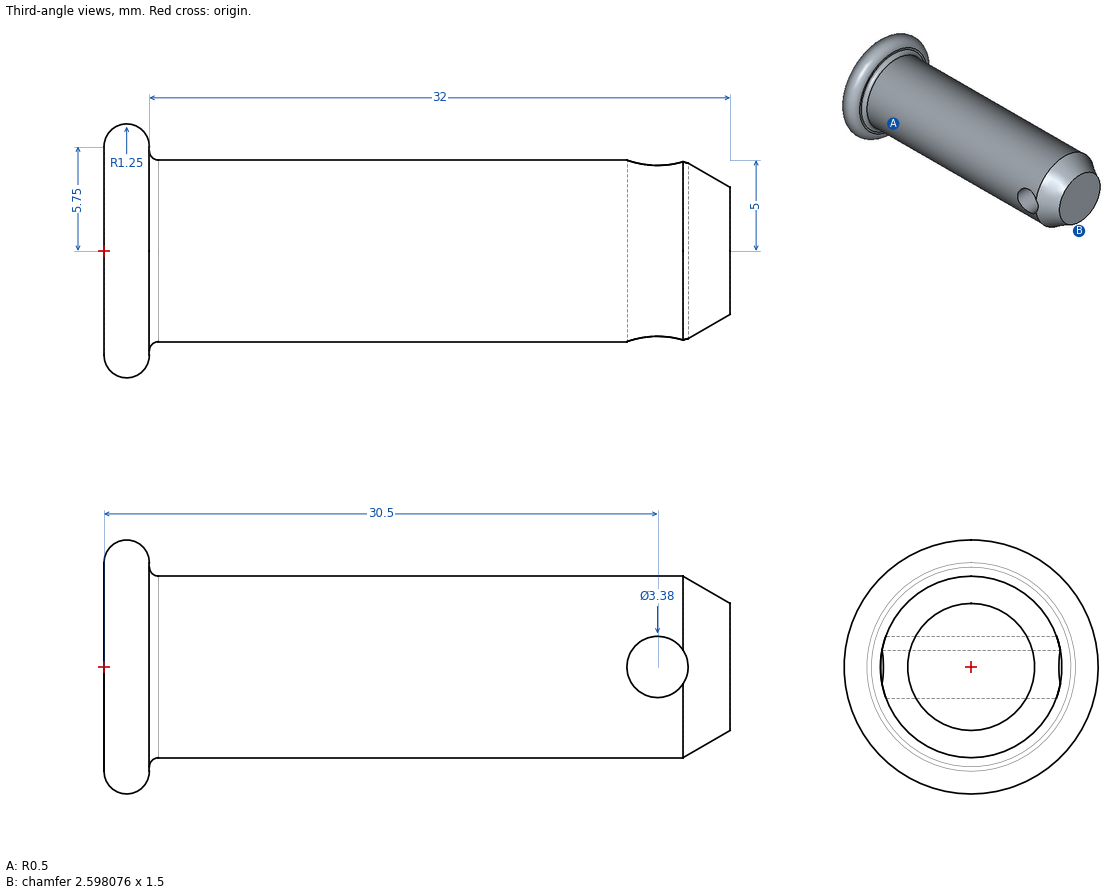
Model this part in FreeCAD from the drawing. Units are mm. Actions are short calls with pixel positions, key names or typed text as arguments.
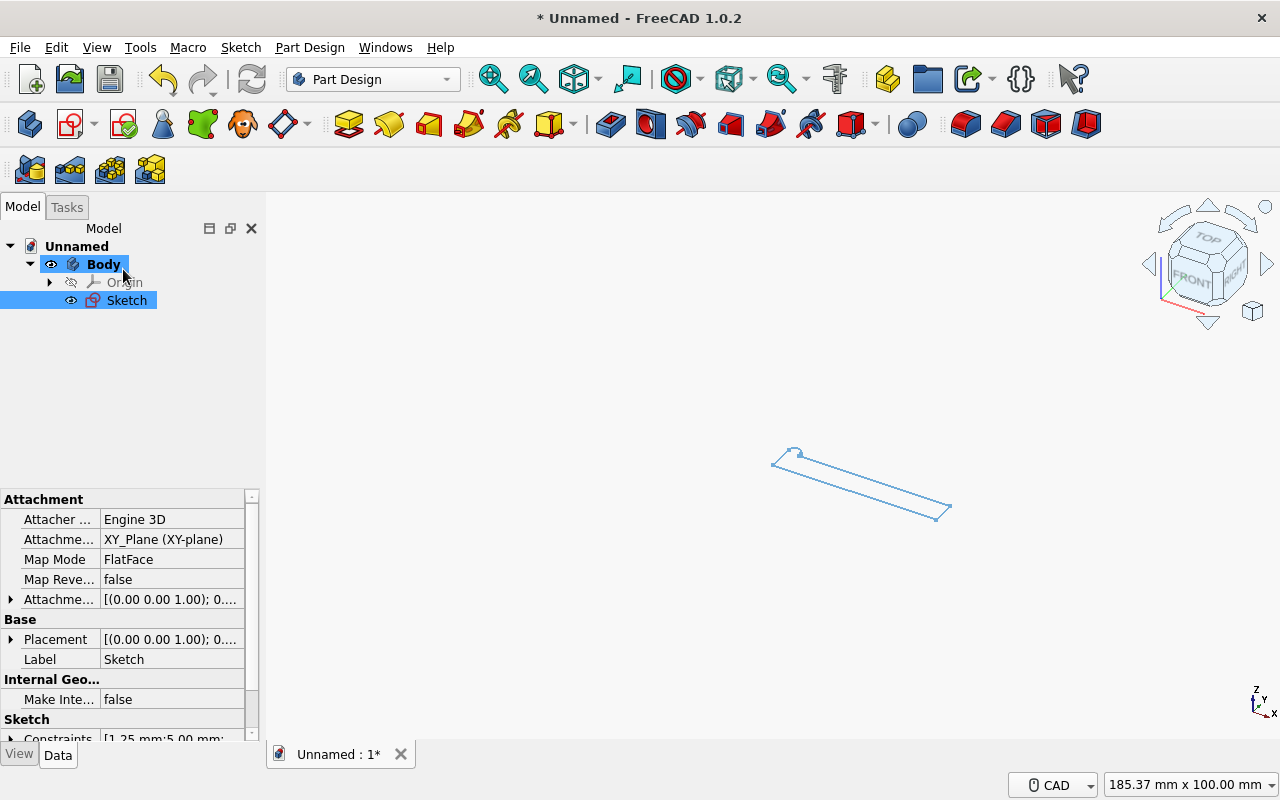
click(390, 124)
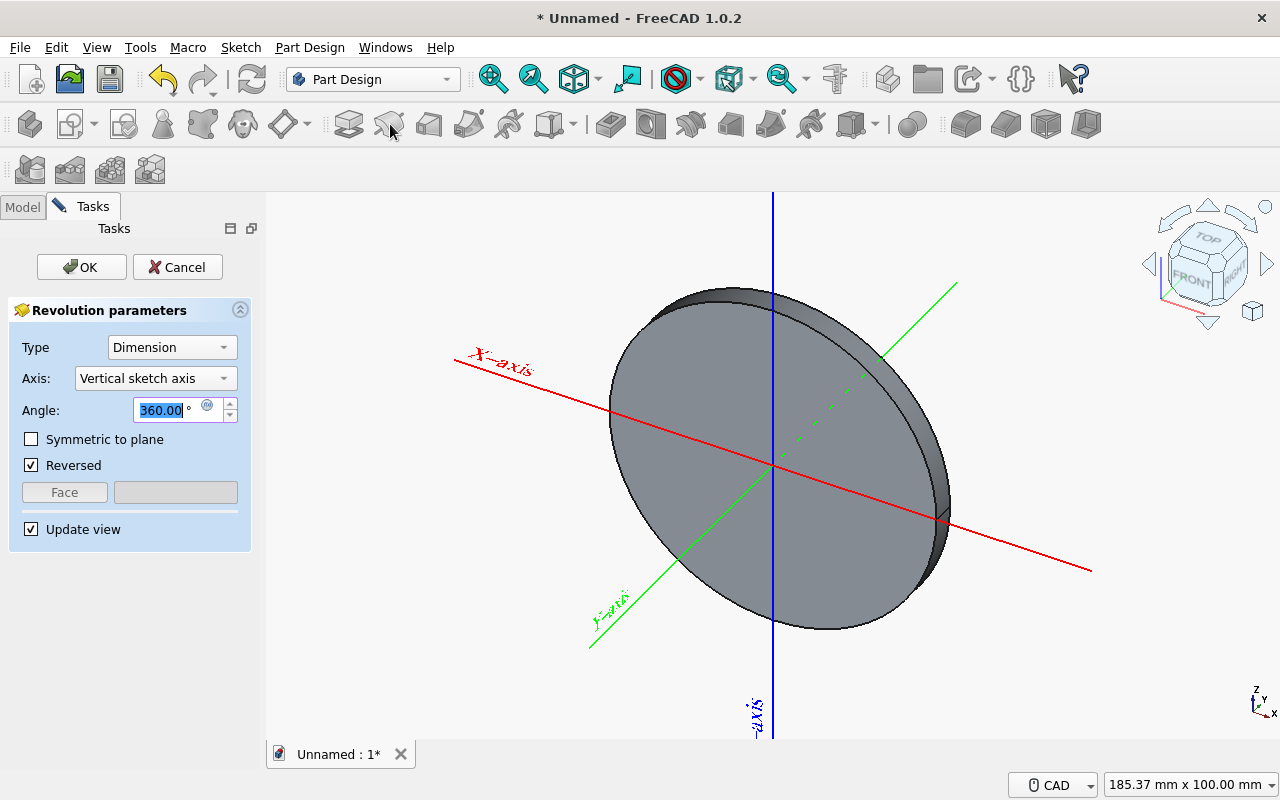
click(156, 378)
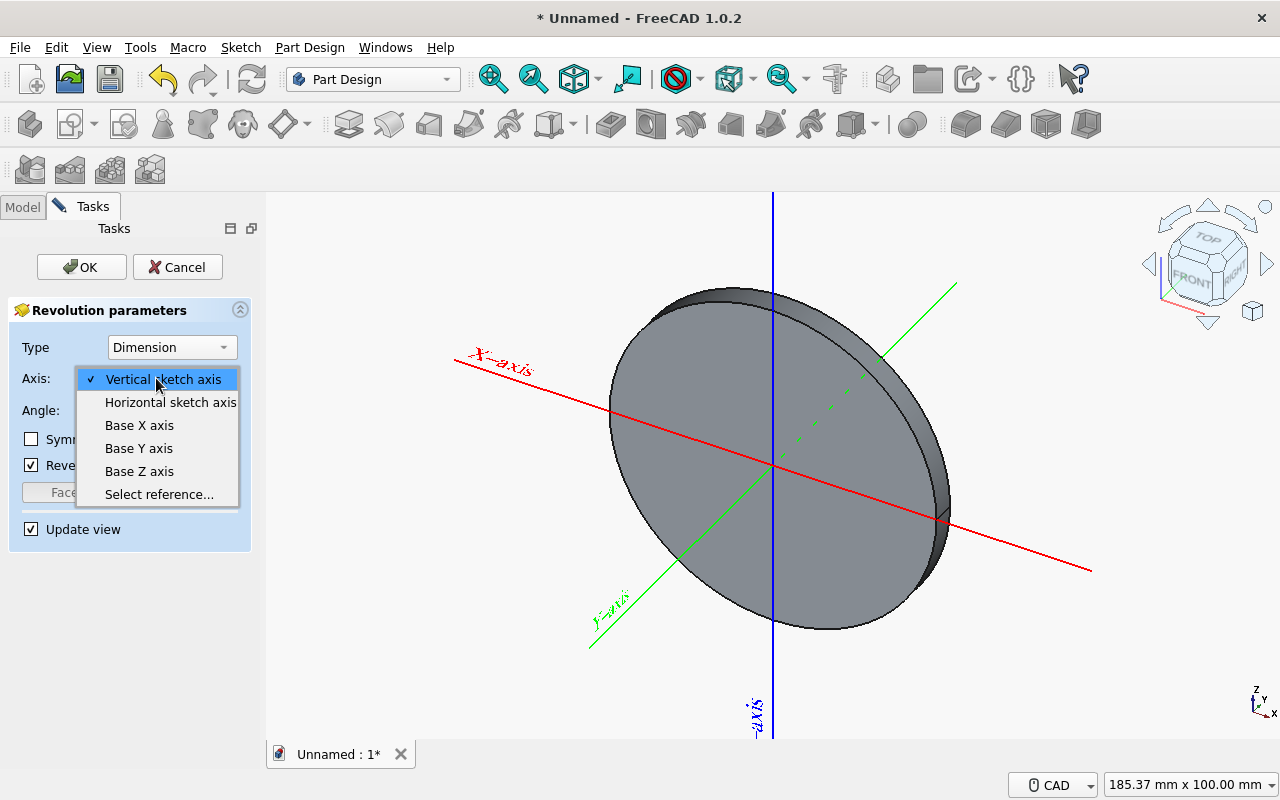
click(156, 402)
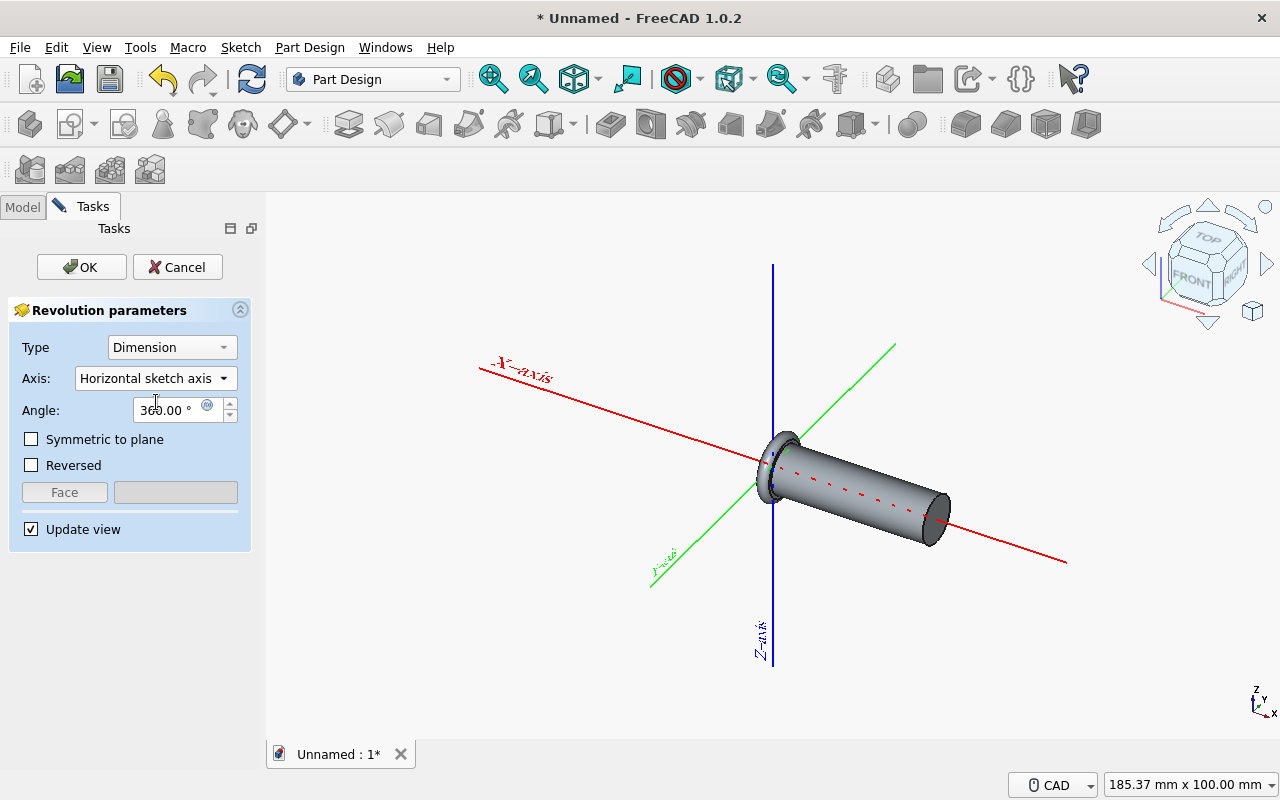
click(82, 267)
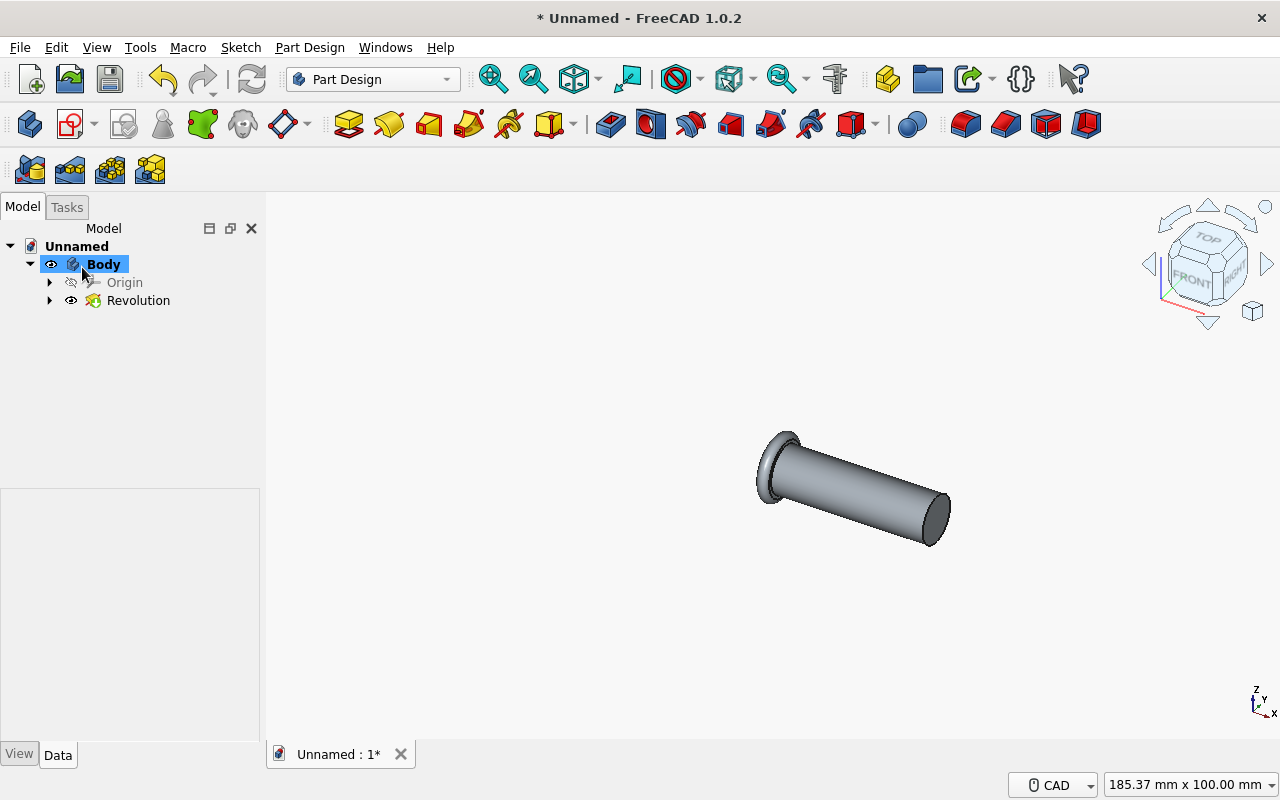
click(494, 80)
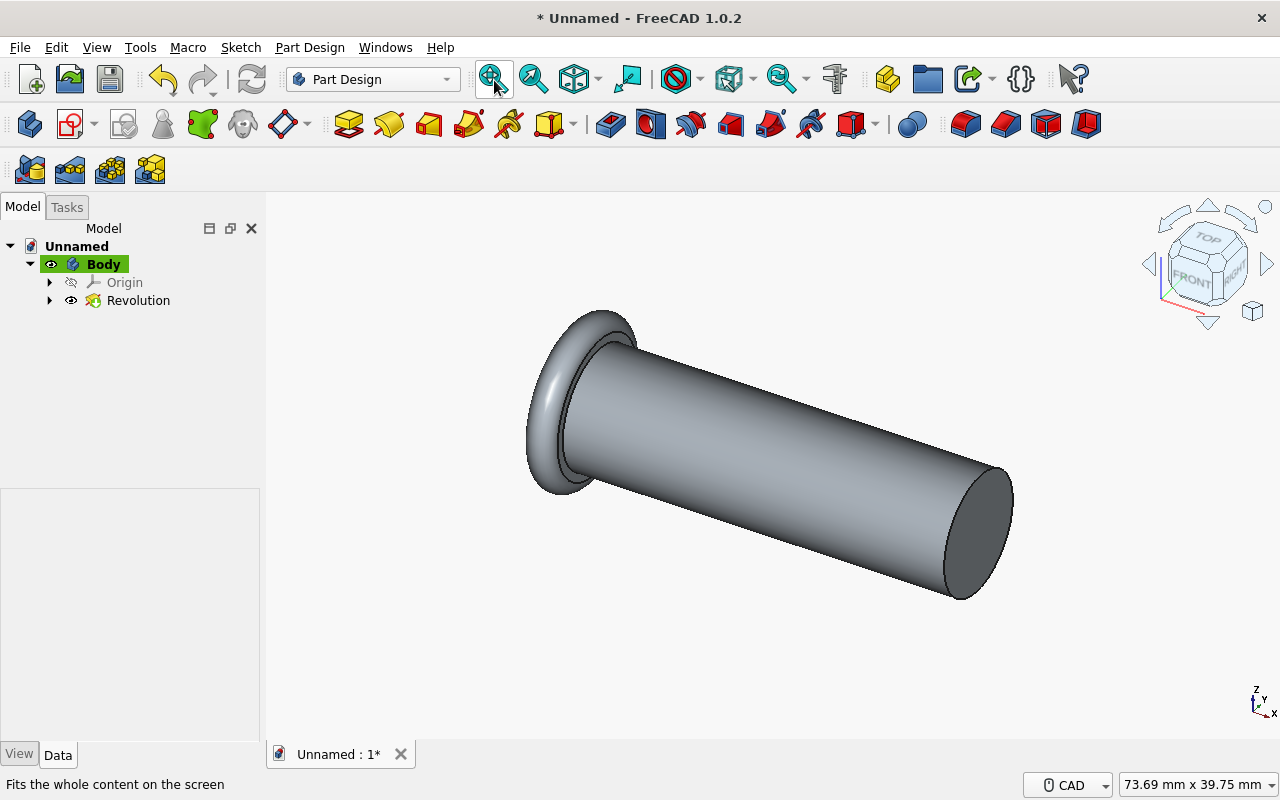
key(0)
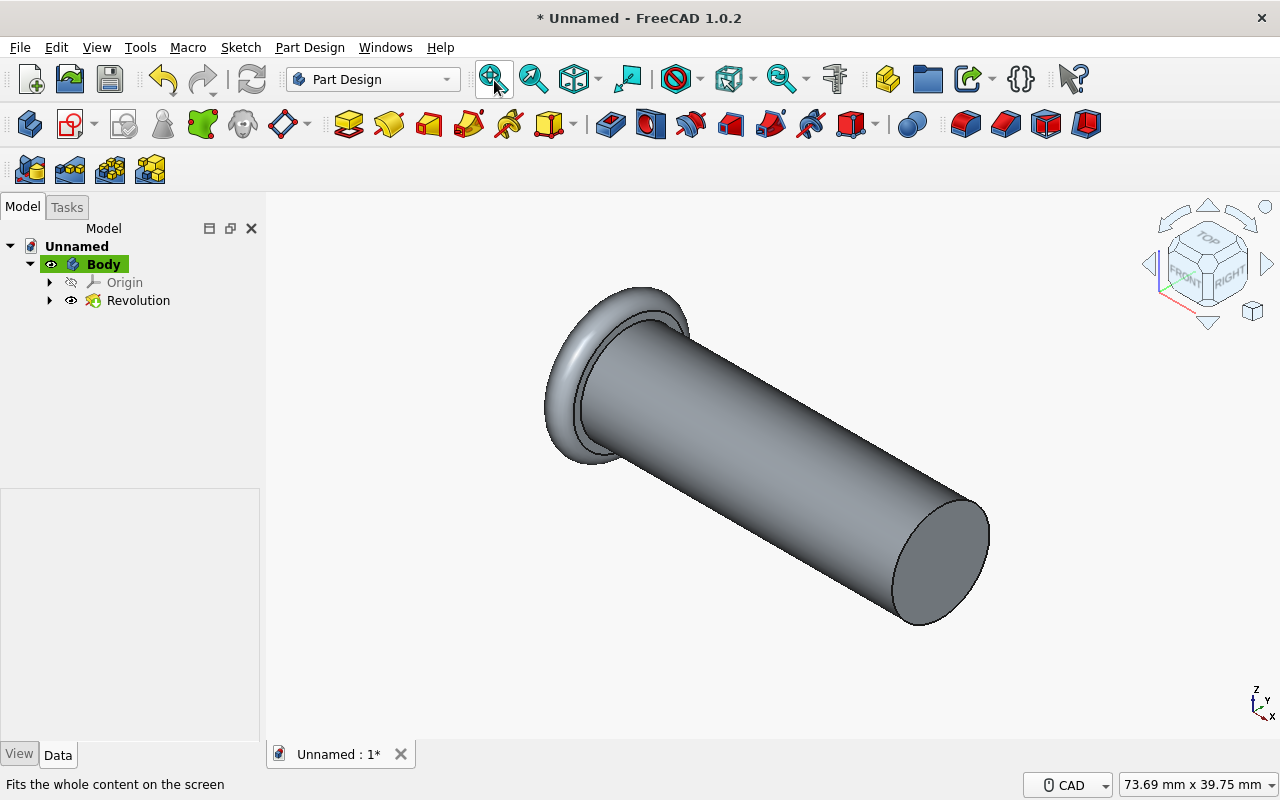
key(2)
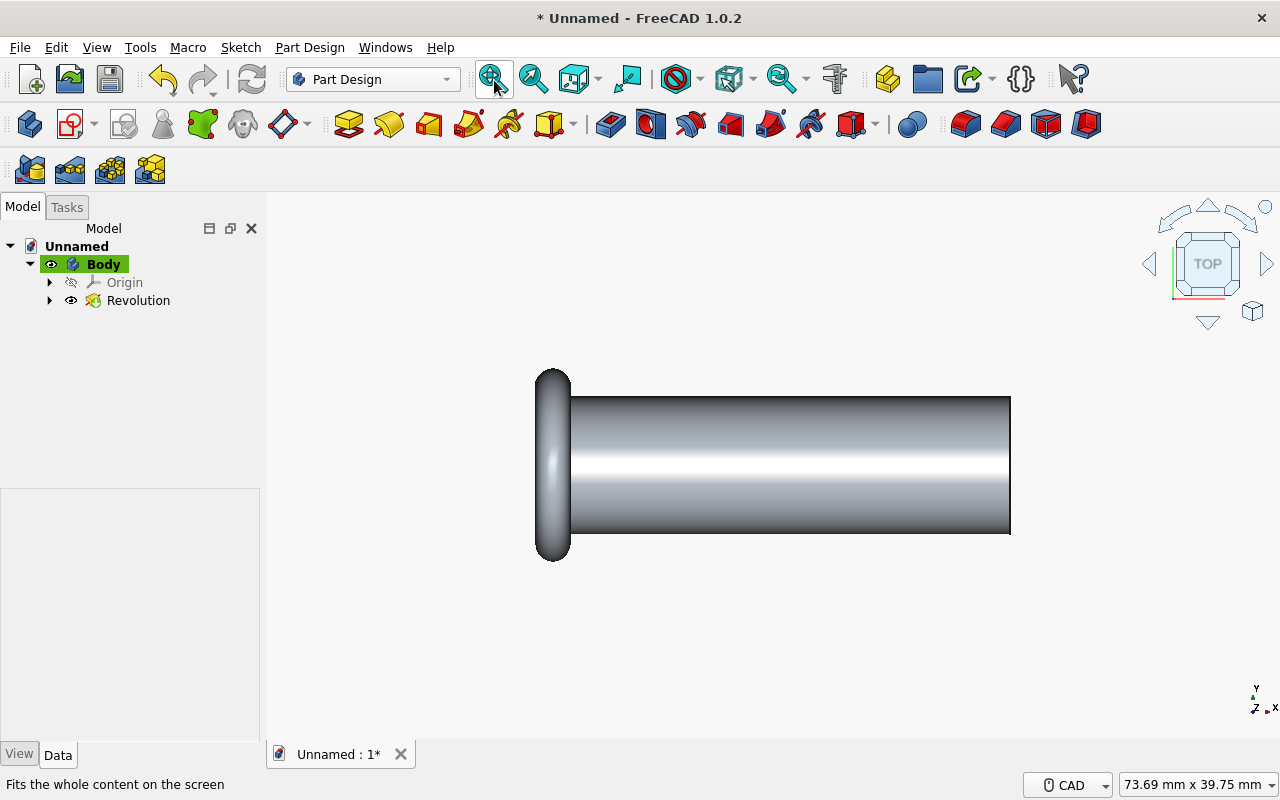
key(1)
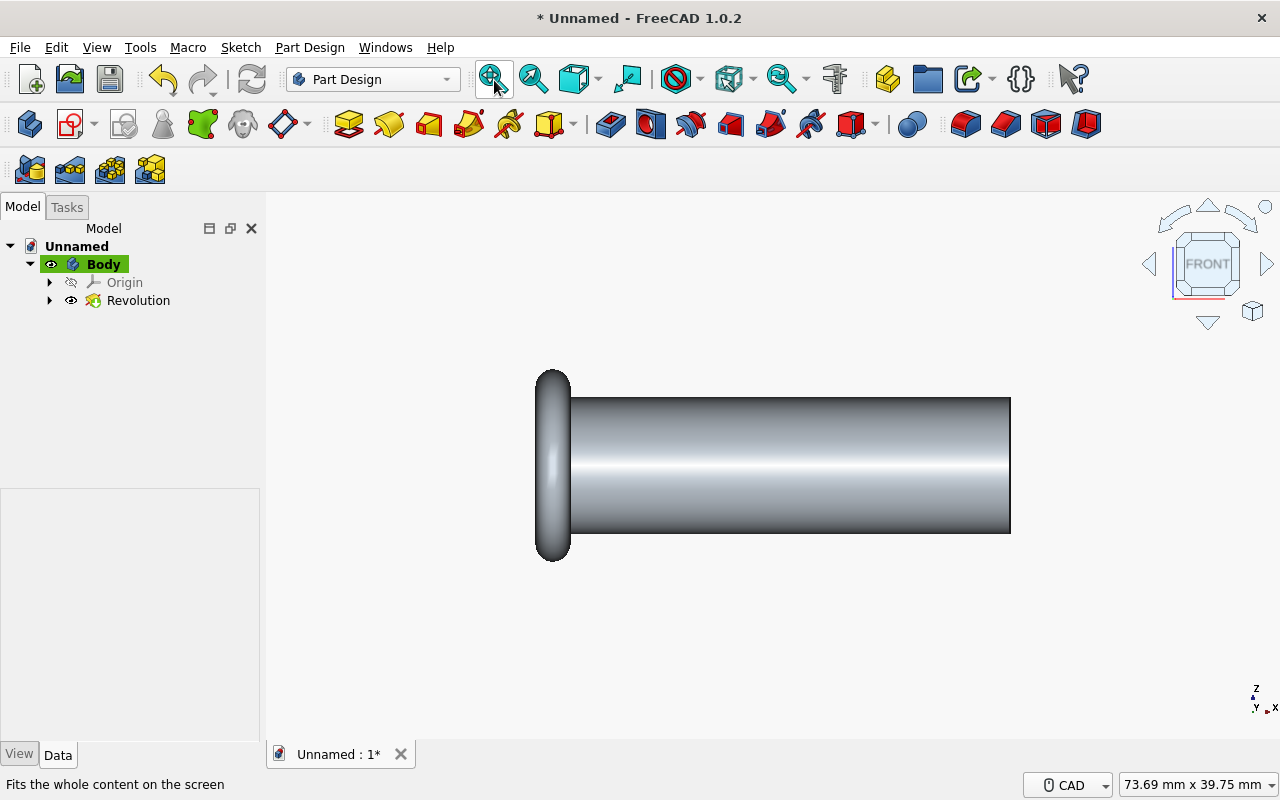
key(3)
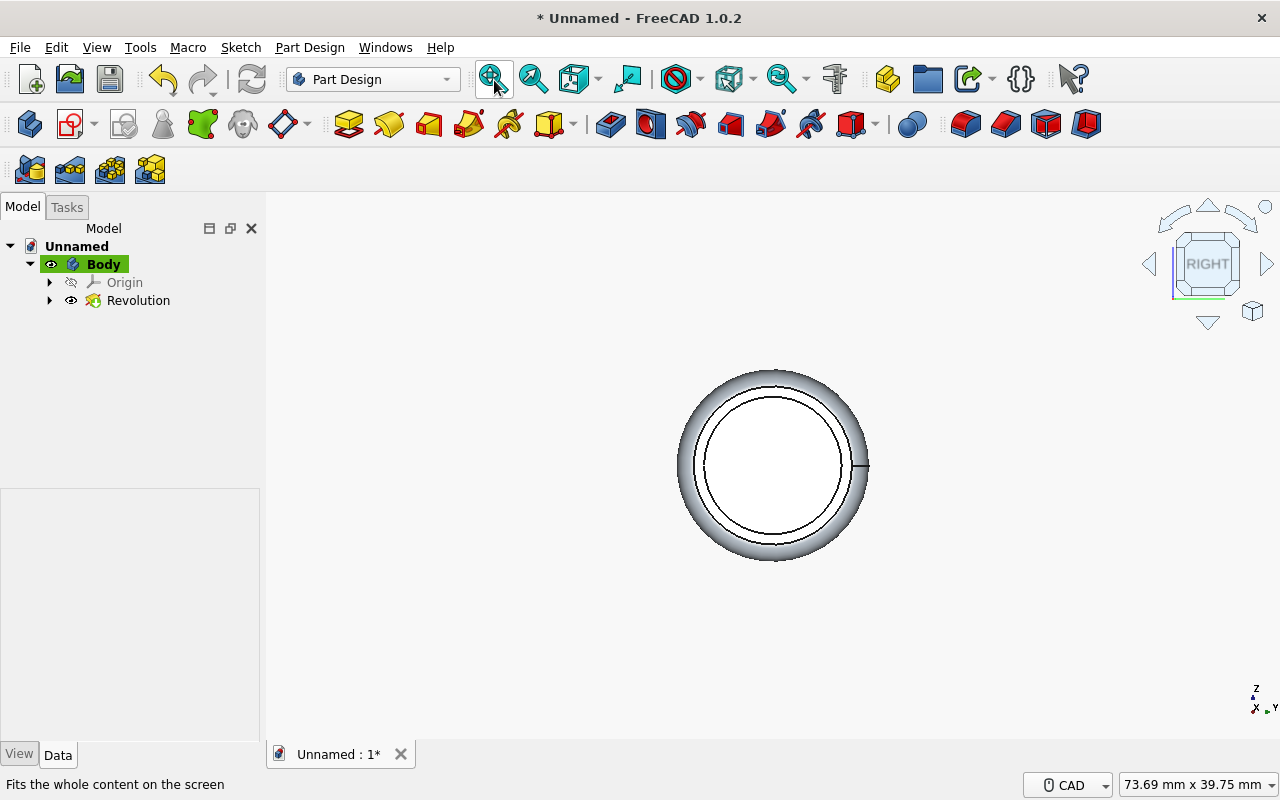
key(v)
key(f)